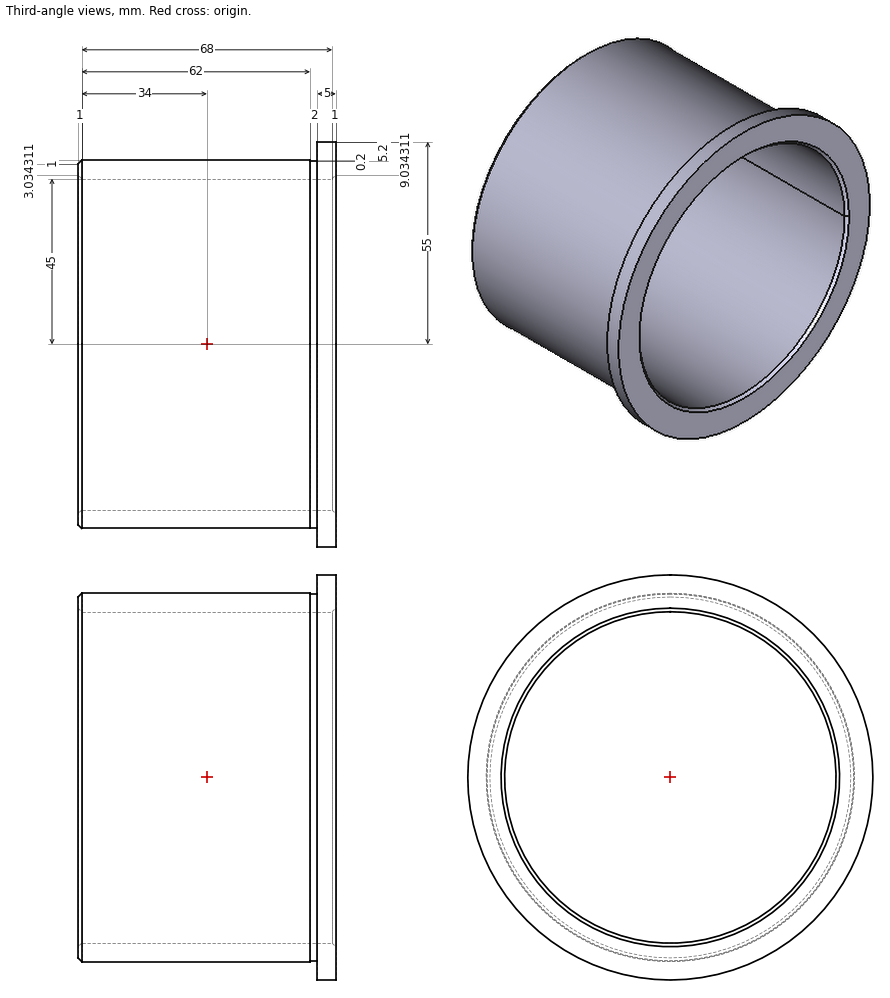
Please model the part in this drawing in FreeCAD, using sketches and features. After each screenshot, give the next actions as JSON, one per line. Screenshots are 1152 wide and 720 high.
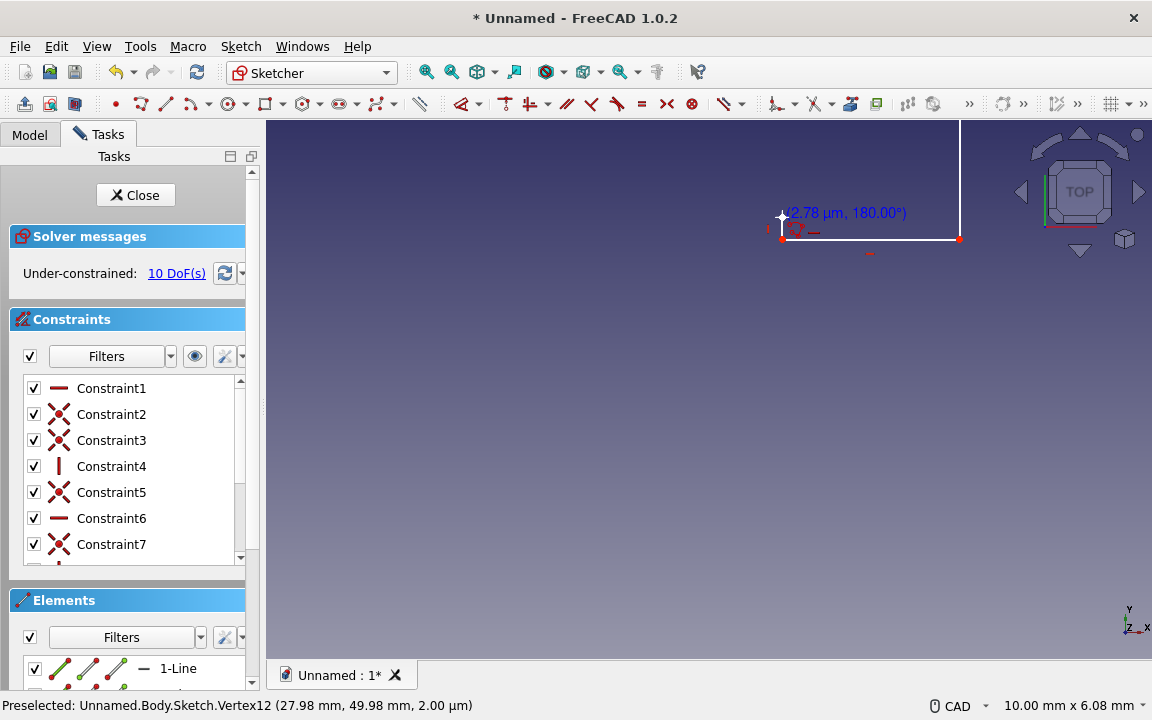
{"action": "scroll", "coordinate": [828, 243], "scroll_direction": "down", "scroll_amount": 13}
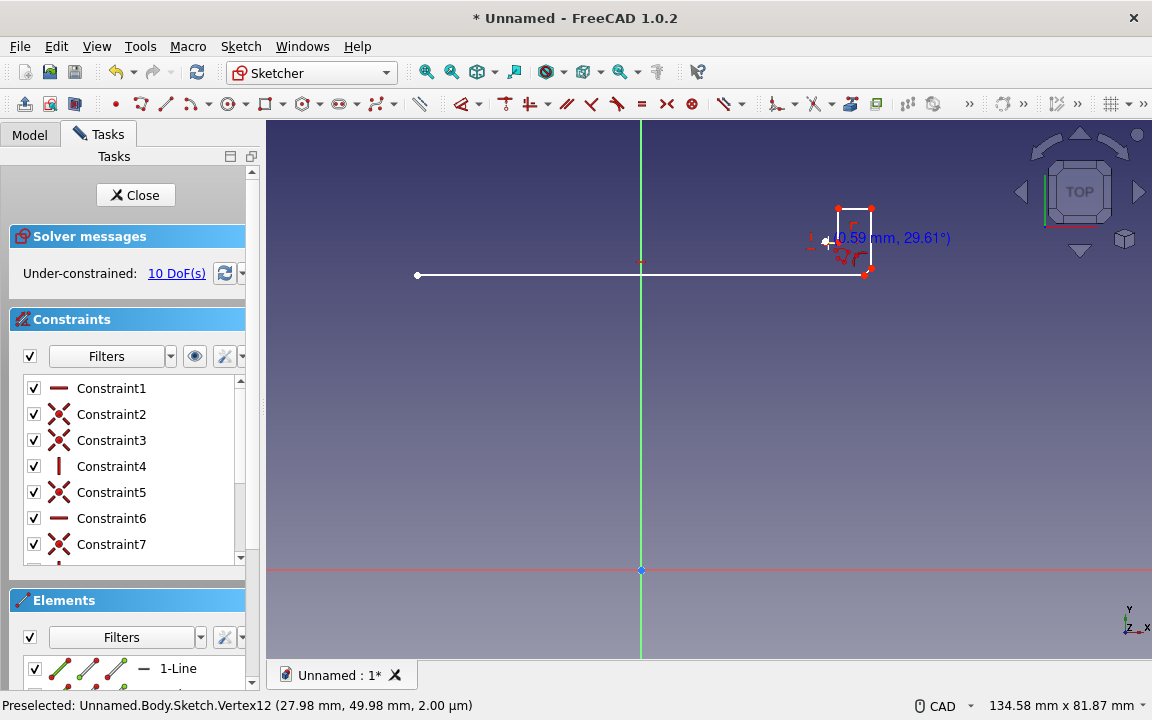
{"action": "left_click", "coordinate": [417, 241]}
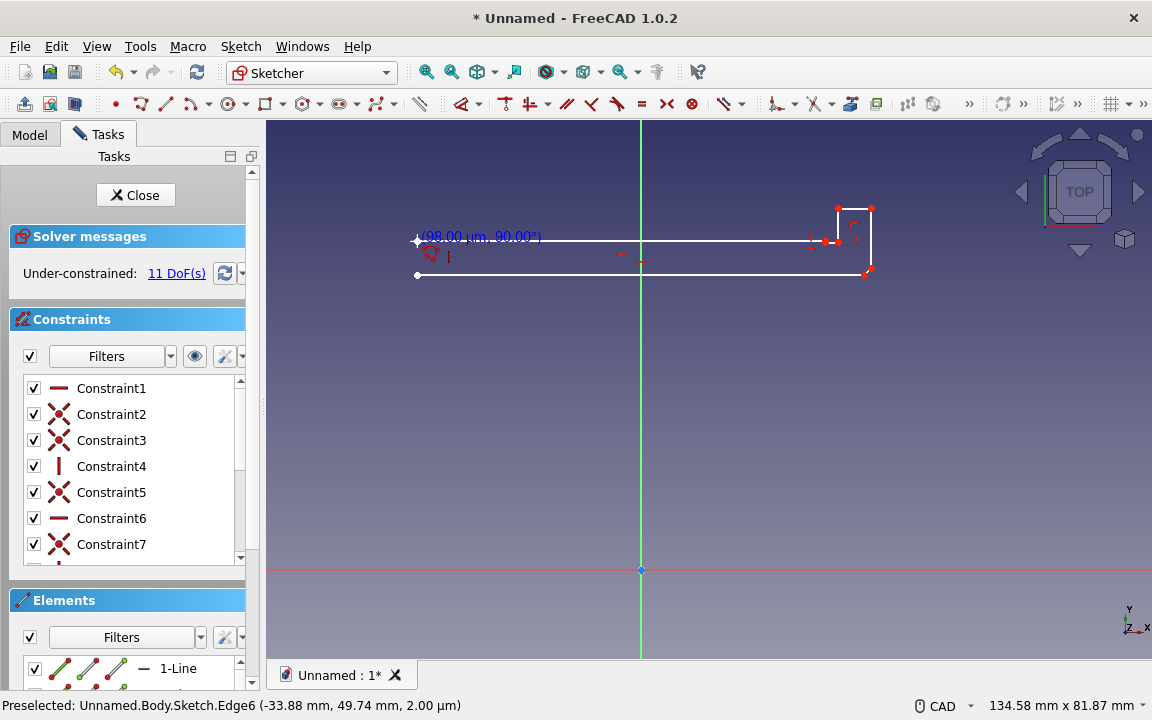
{"action": "scroll", "coordinate": [411, 248], "scroll_direction": "up", "scroll_amount": 3}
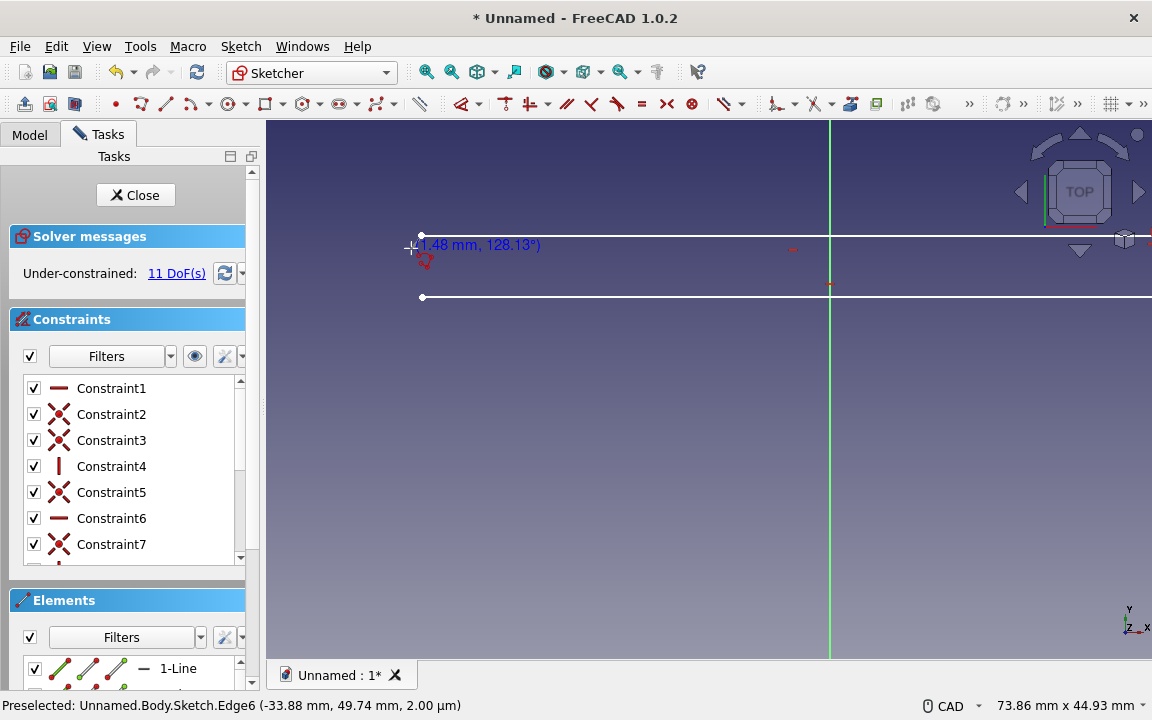
{"action": "left_click", "coordinate": [410, 248]}
{"action": "left_click", "coordinate": [410, 284]}
{"action": "left_click", "coordinate": [423, 297]}
{"action": "key", "text": "Escape"}
{"action": "key", "text": "Escape"}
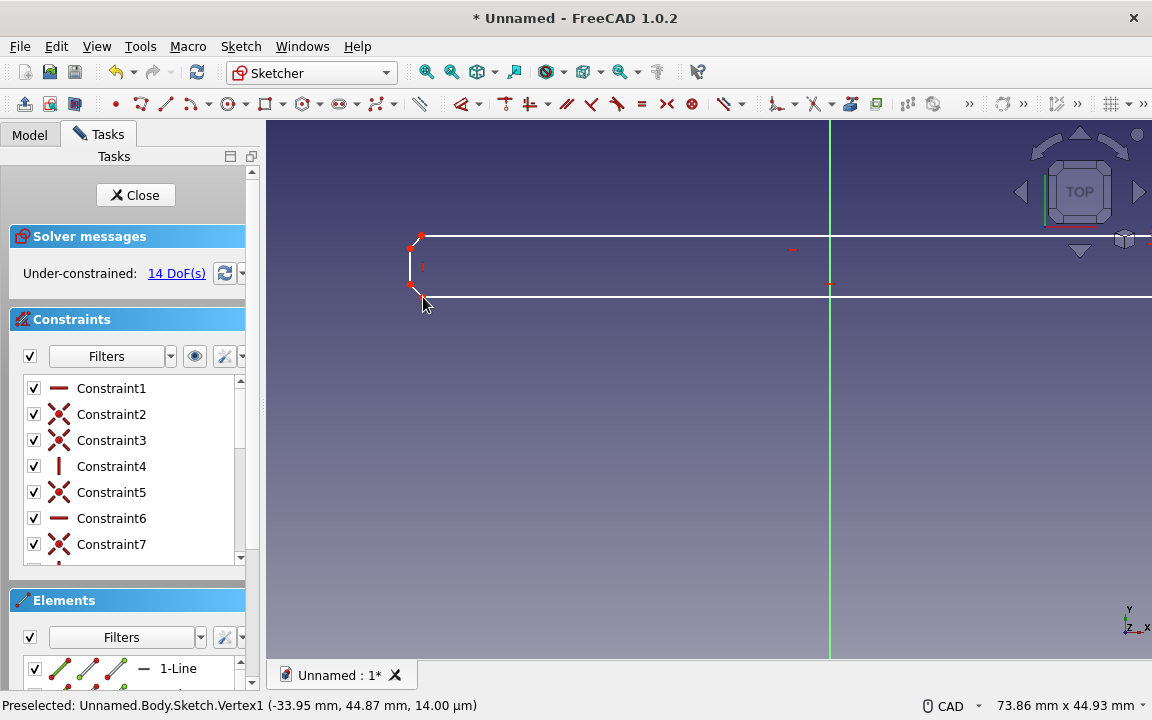
{"action": "scroll", "coordinate": [410, 248], "scroll_direction": "down", "scroll_amount": 3}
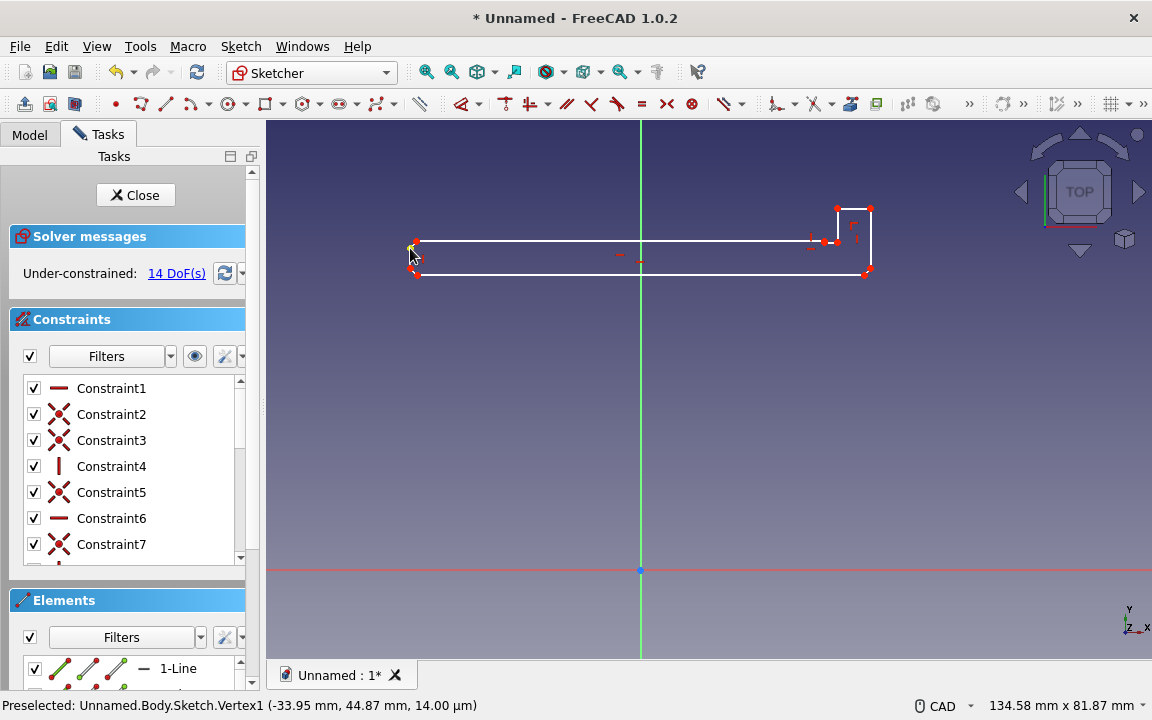
{"action": "scroll", "coordinate": [861, 209], "scroll_direction": "up", "scroll_amount": 2}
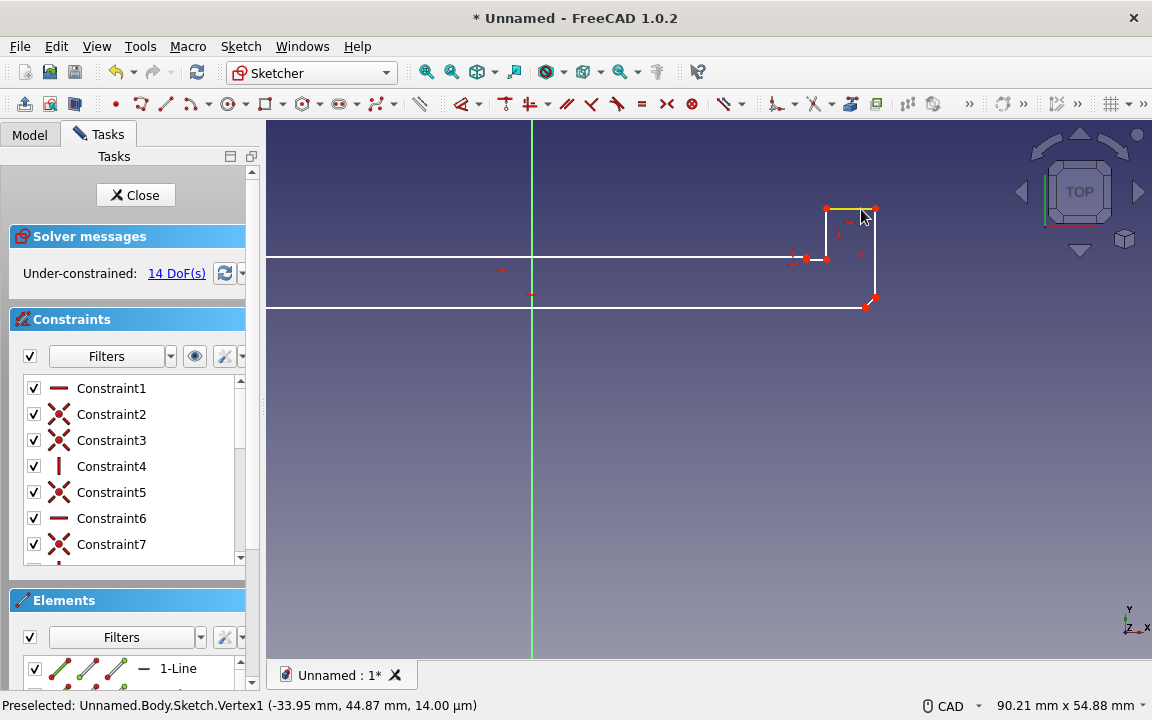
{"action": "left_click", "coordinate": [861, 209]}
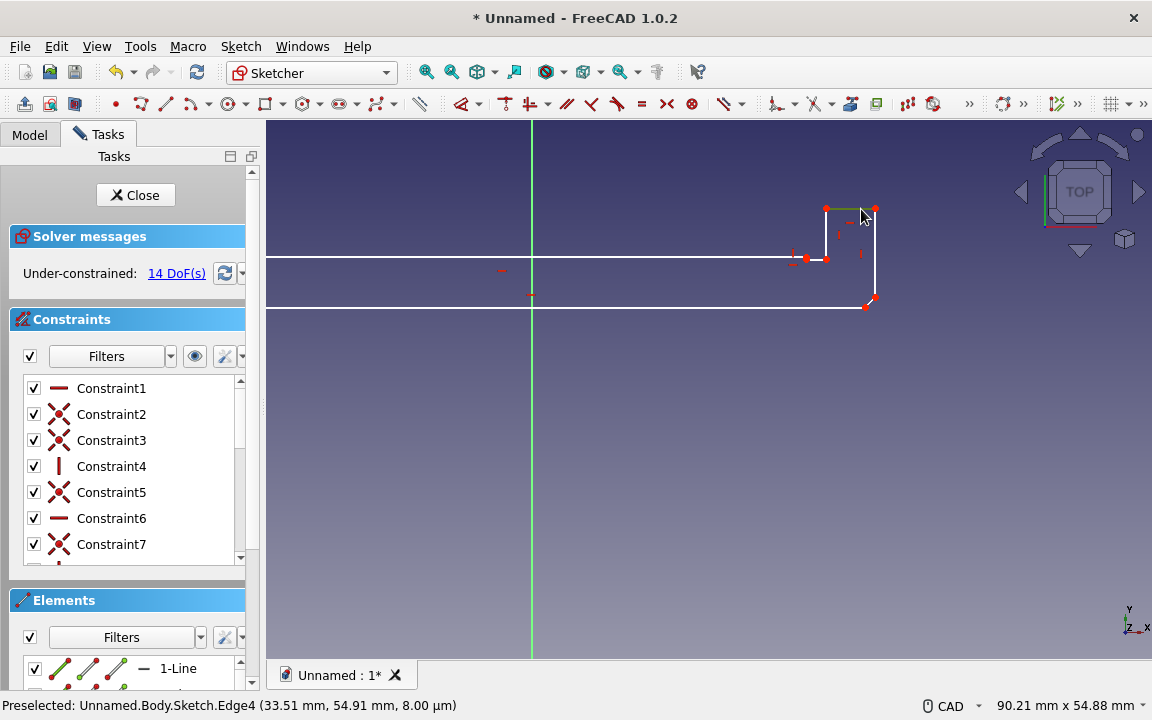
{"action": "left_click", "coordinate": [478, 104]}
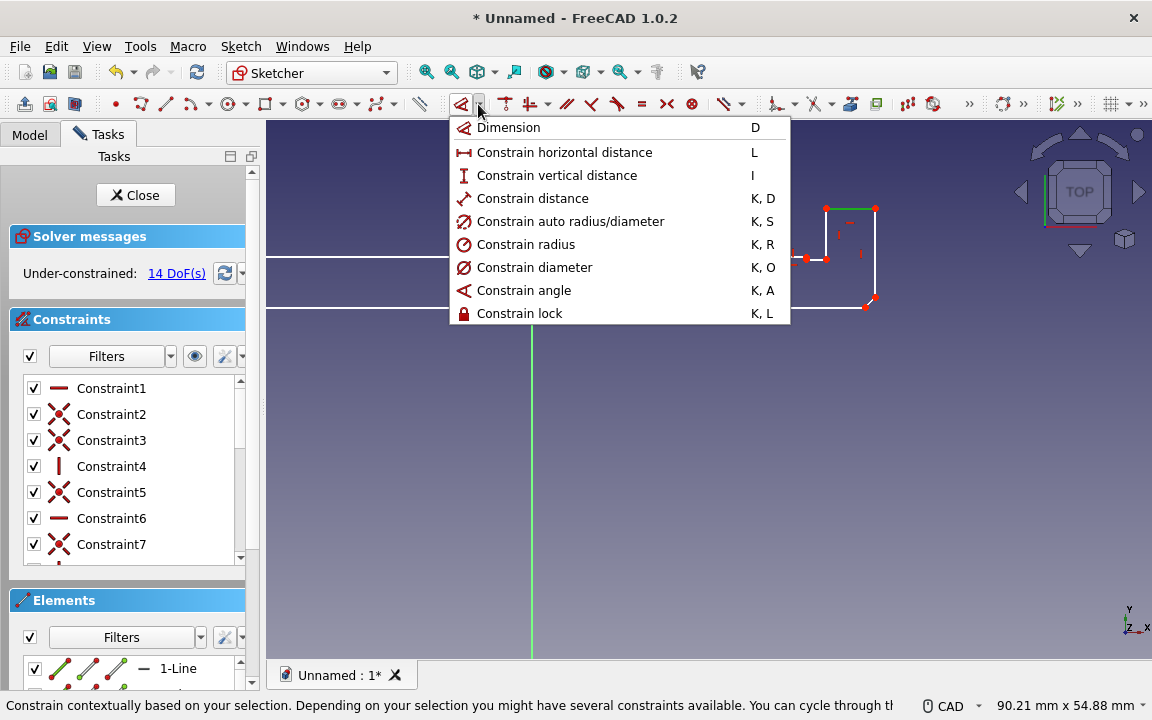
{"action": "left_click", "coordinate": [620, 152]}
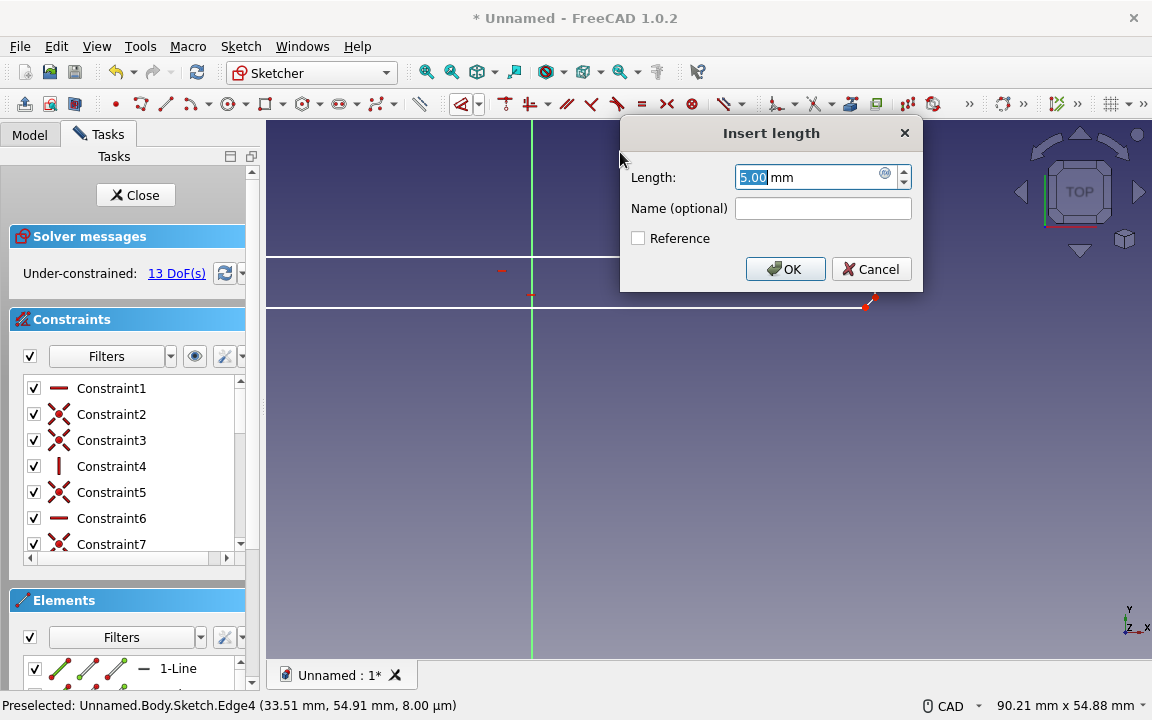
{"action": "type", "text": "5"}
{"action": "key", "text": "Return"}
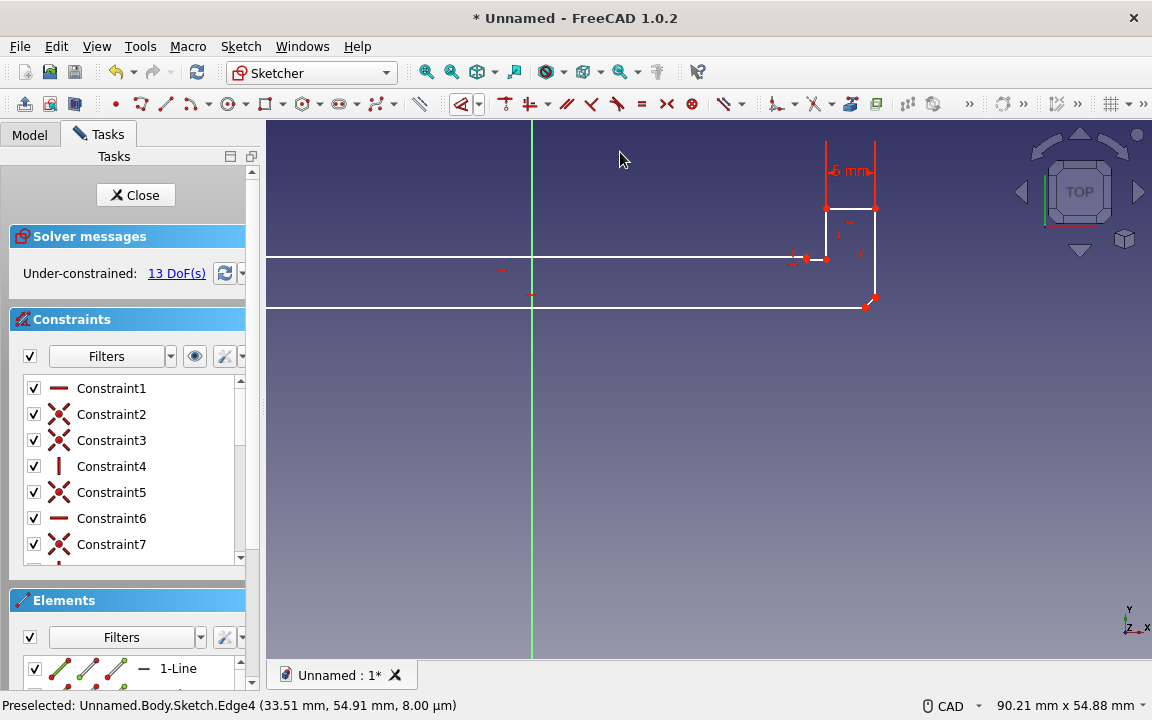
{"action": "scroll", "coordinate": [816, 260], "scroll_direction": "up", "scroll_amount": 4}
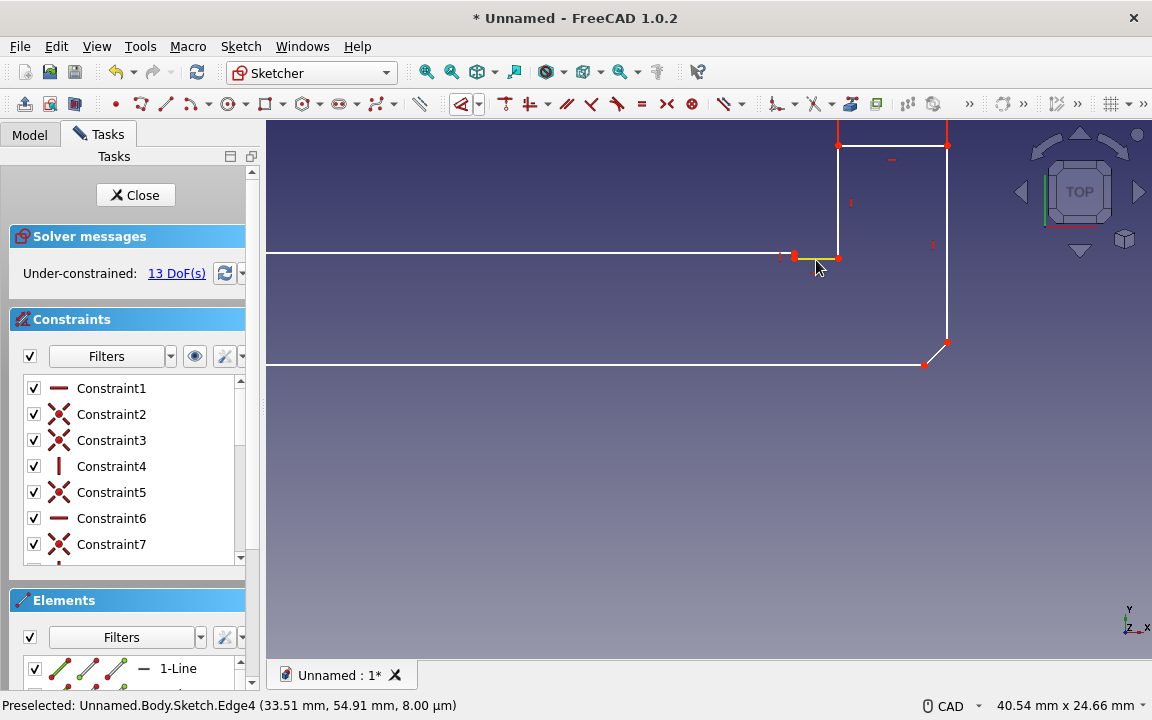
{"action": "left_click", "coordinate": [816, 259]}